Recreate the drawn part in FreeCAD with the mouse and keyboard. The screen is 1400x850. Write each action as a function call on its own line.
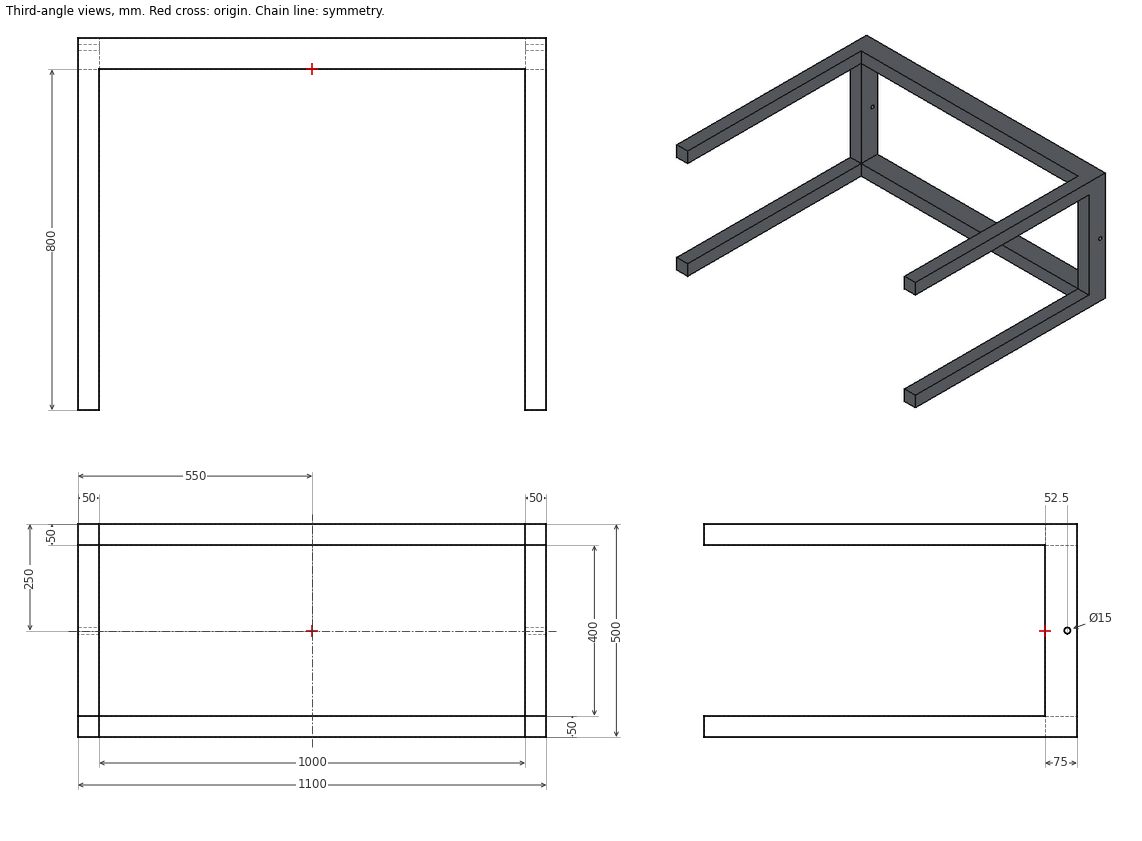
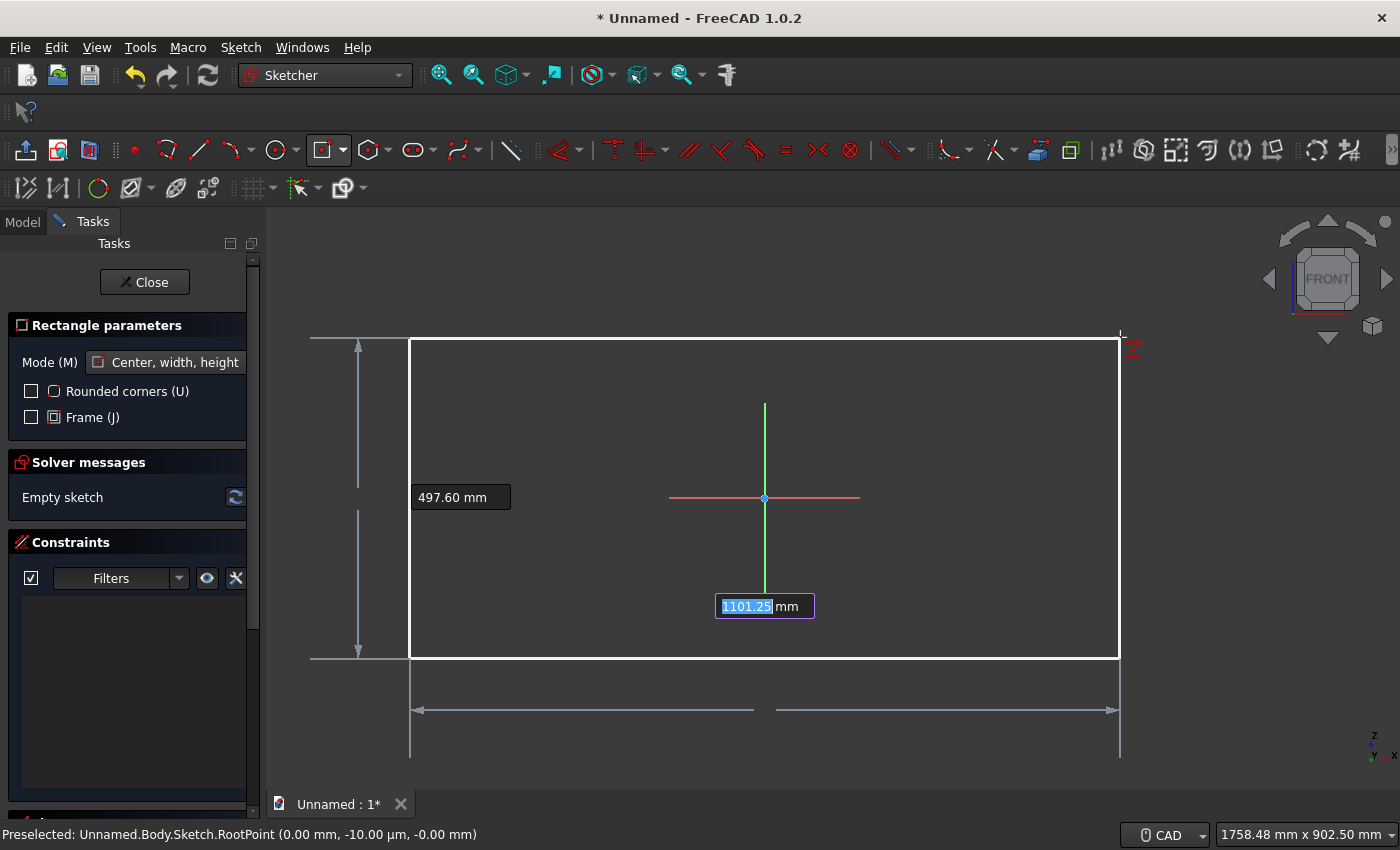
text(1100)
key(Tab)
text(500)
key(Return)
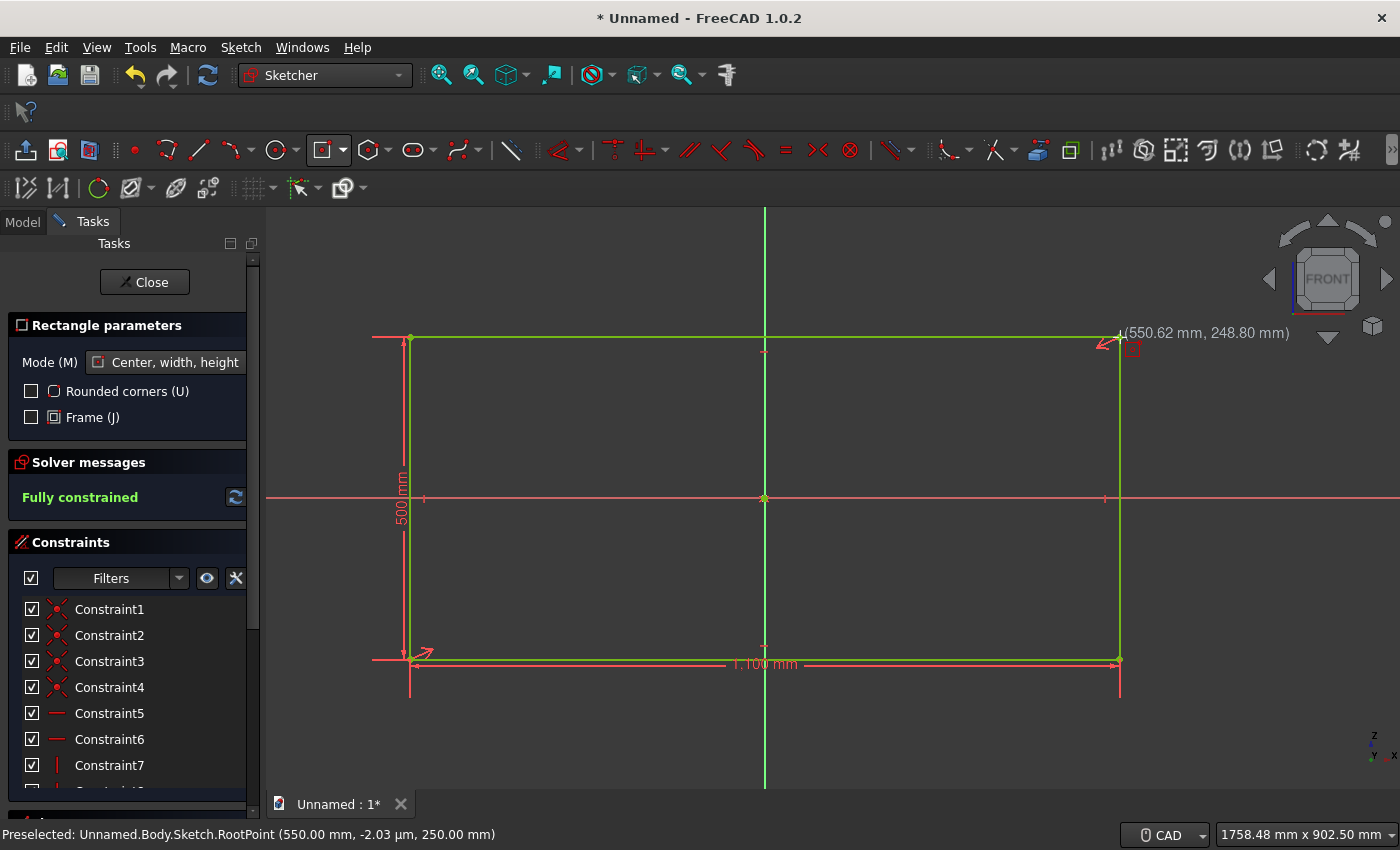
click(765, 498)
move(1087, 369)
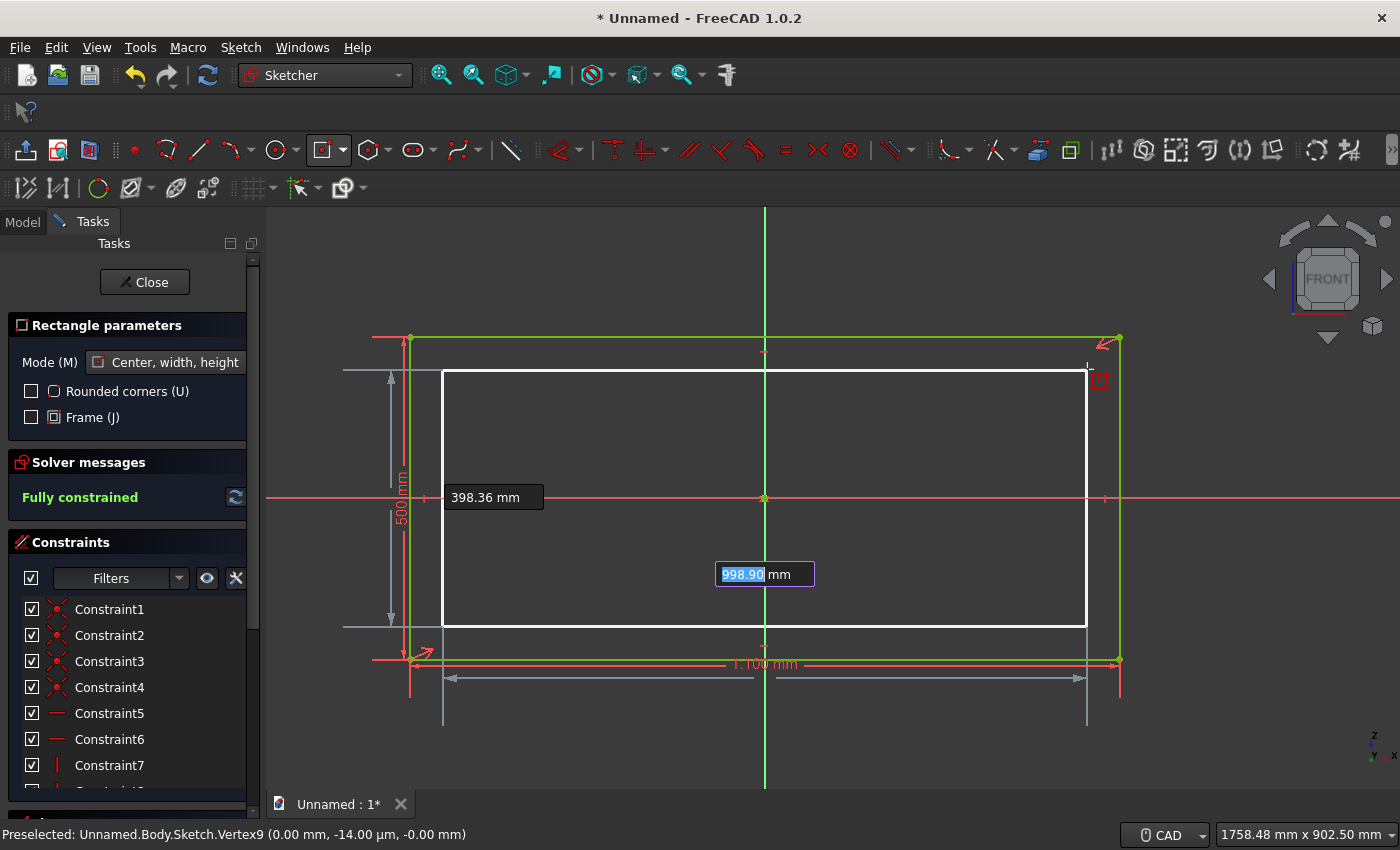
text(1000)
key(Tab)
text(400)
key(Return)
key(Escape)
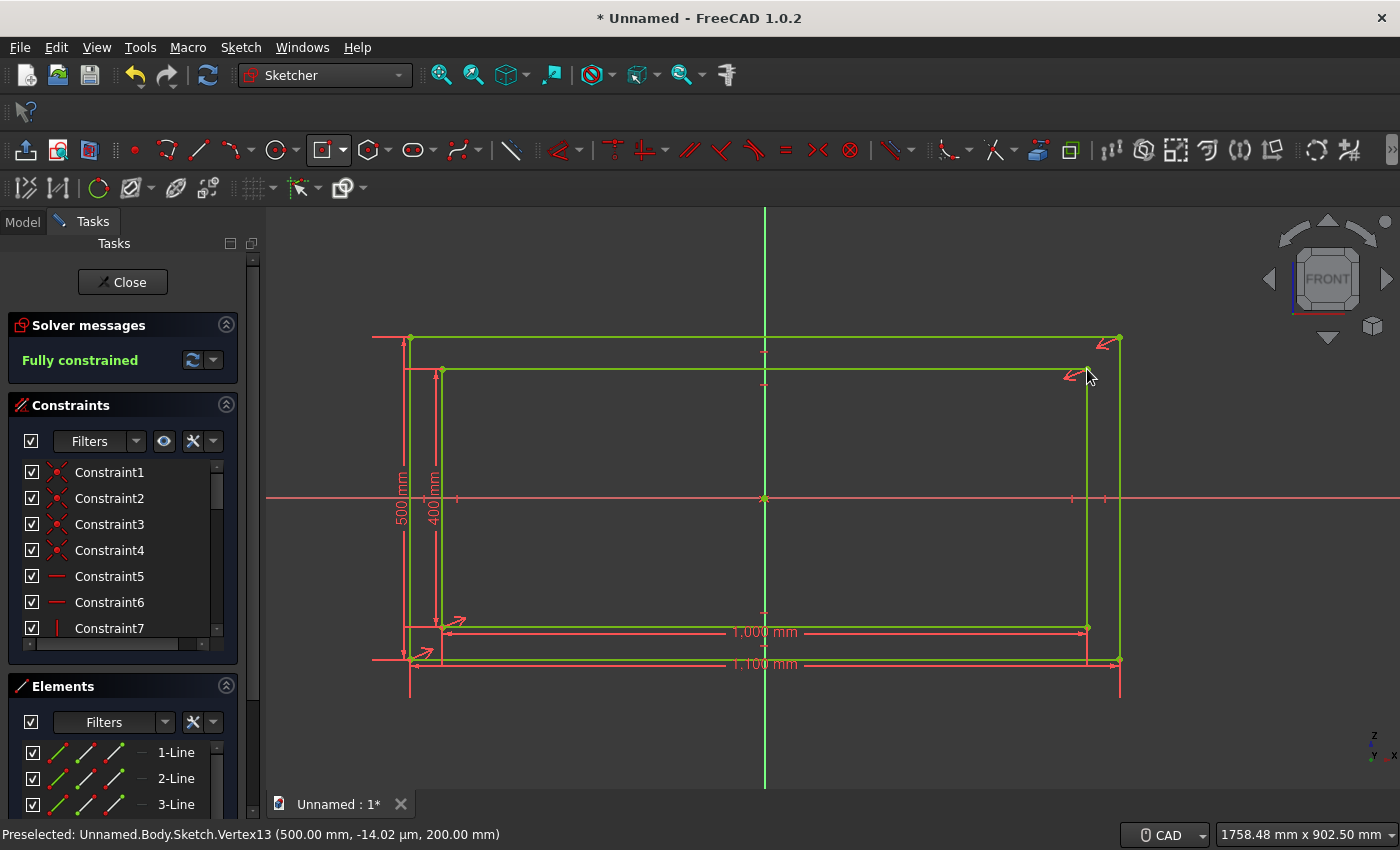
click(123, 282)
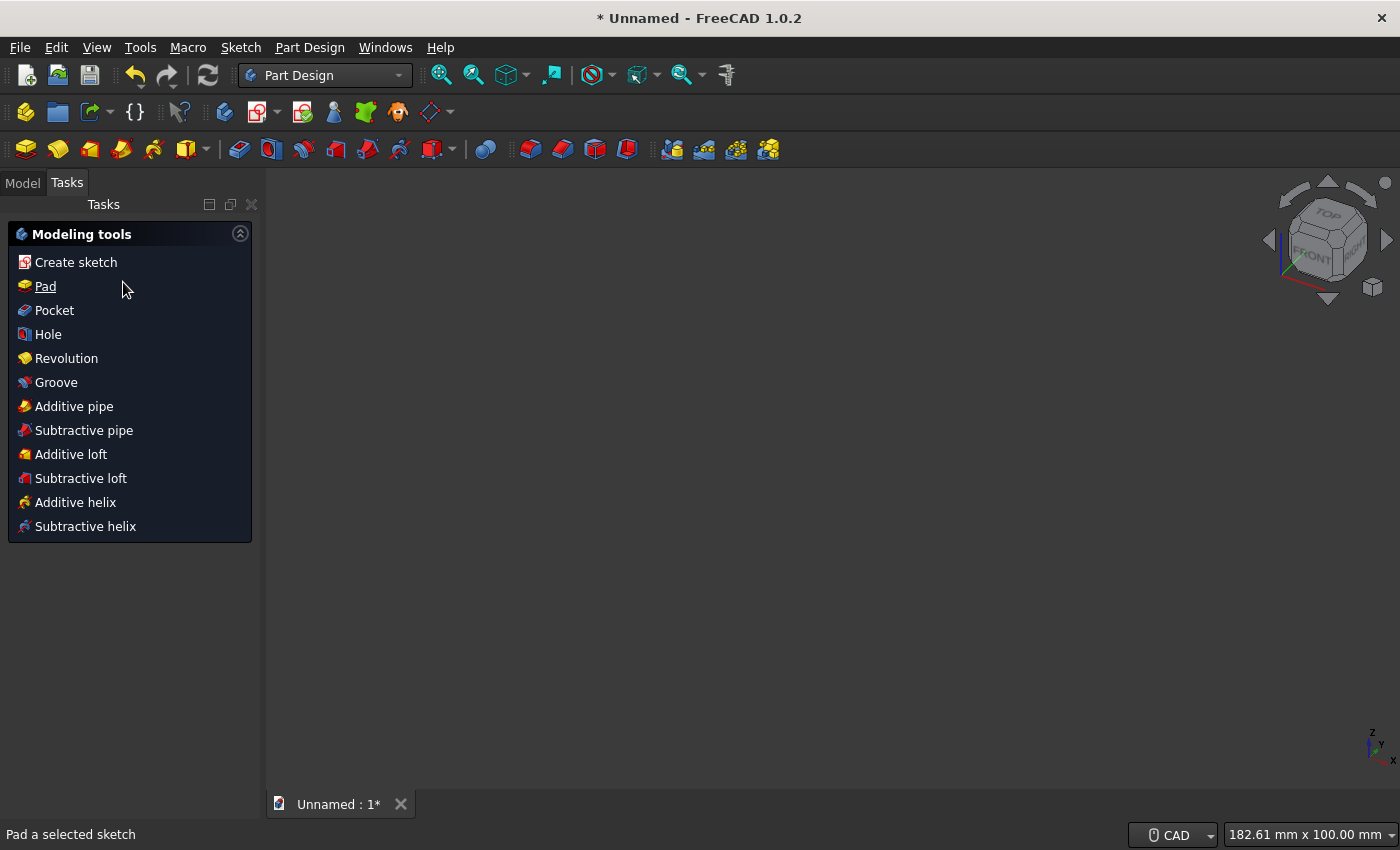
click(26, 150)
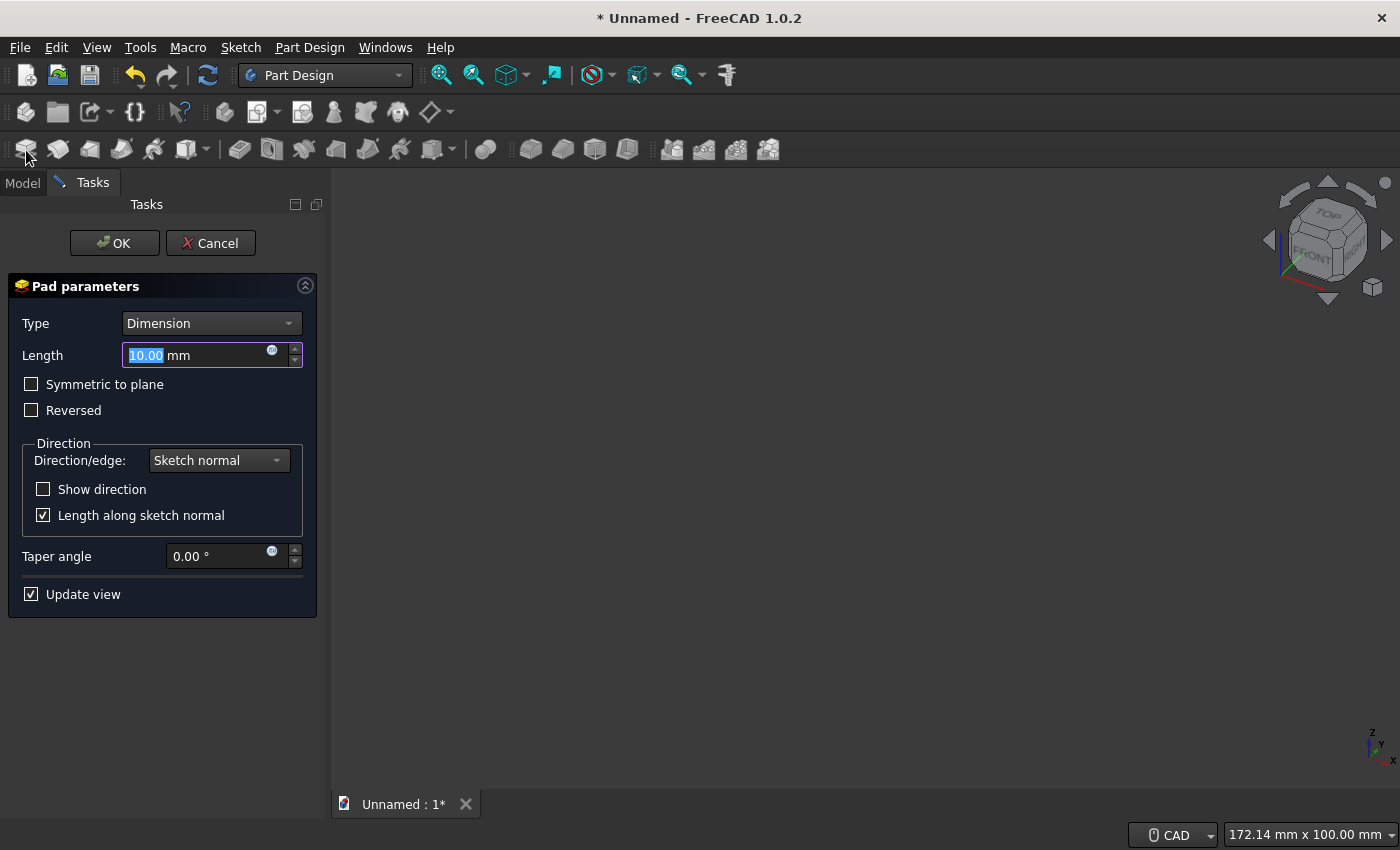
text(75)
key(Tab)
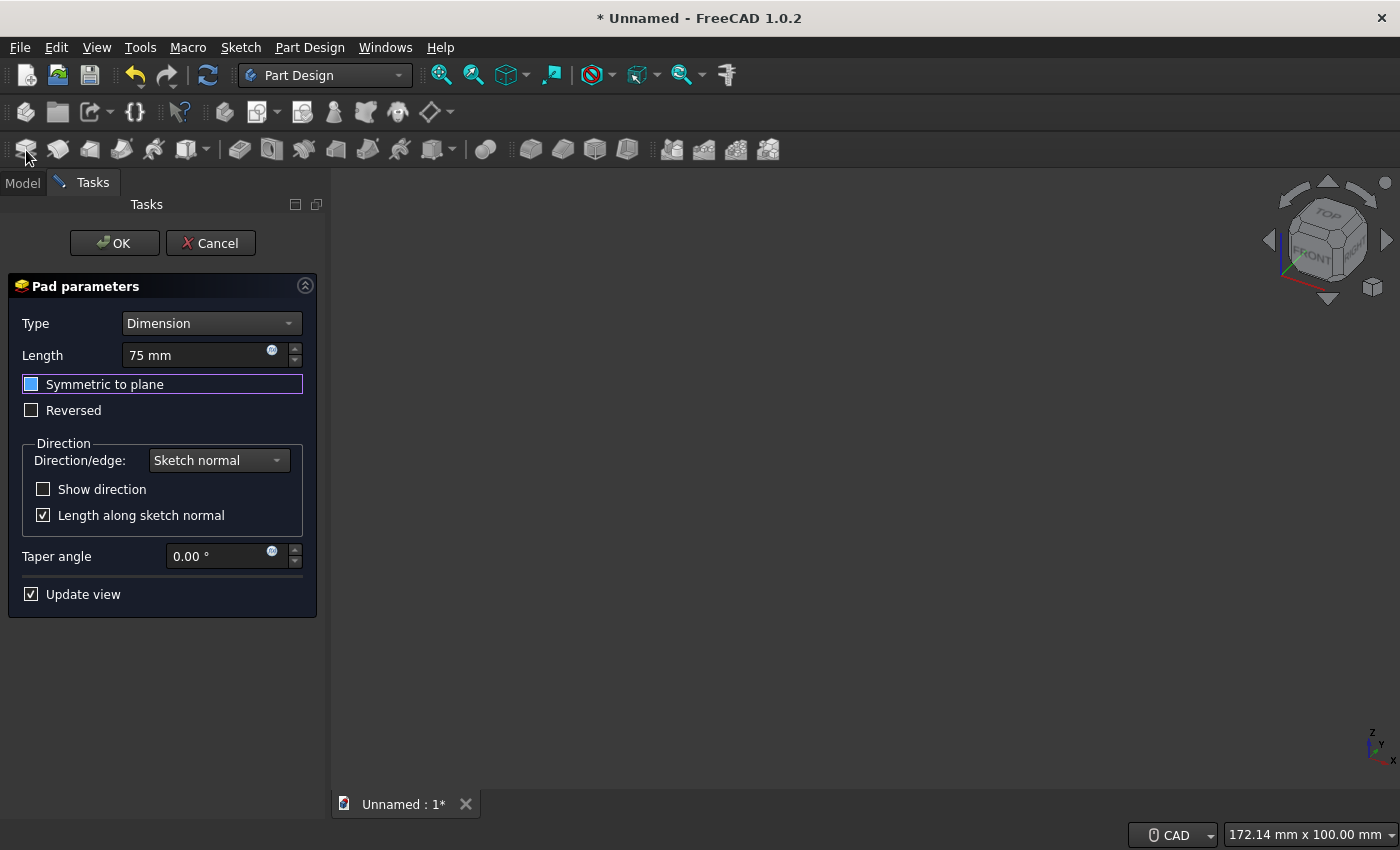
click(30, 410)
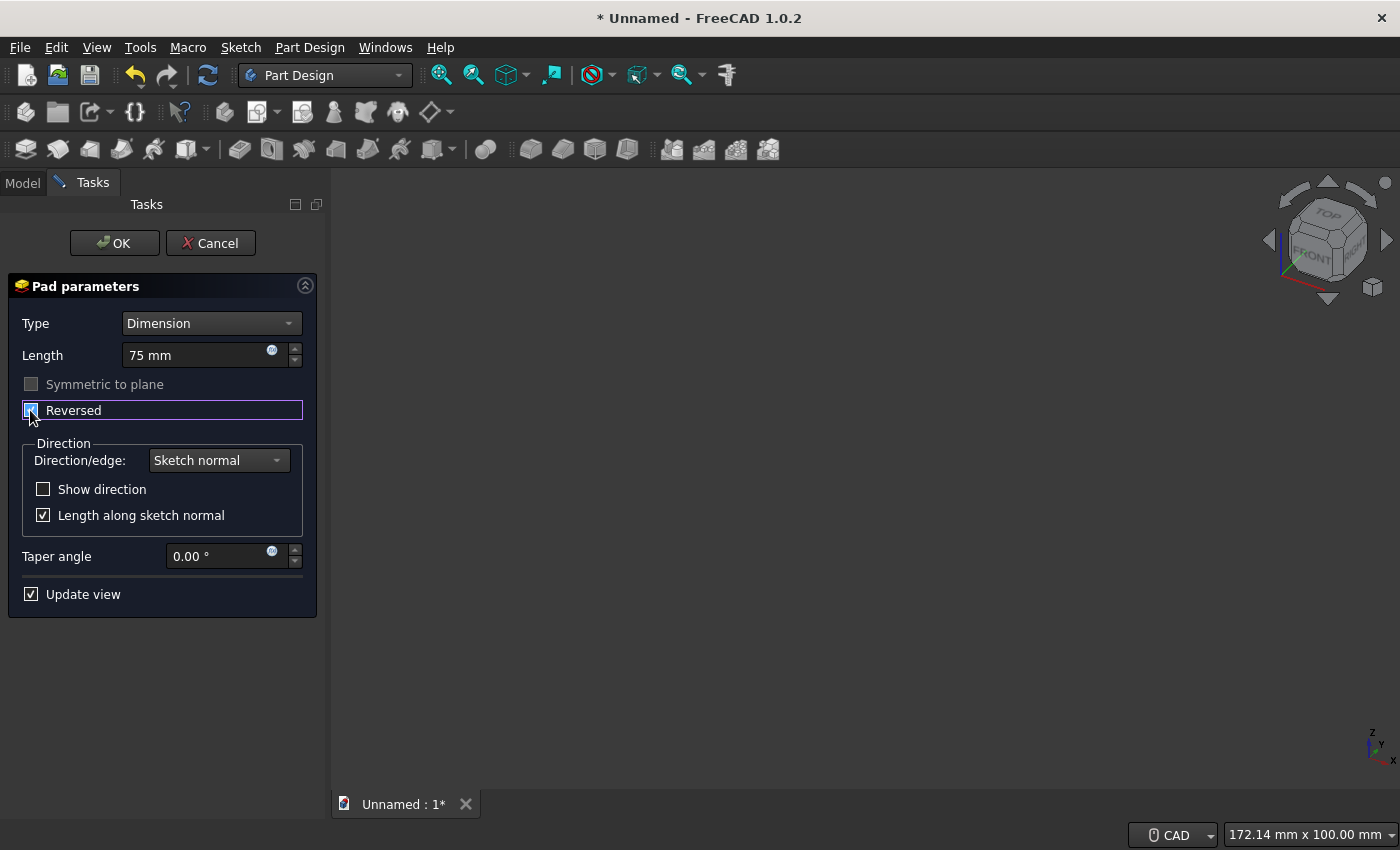
click(115, 243)